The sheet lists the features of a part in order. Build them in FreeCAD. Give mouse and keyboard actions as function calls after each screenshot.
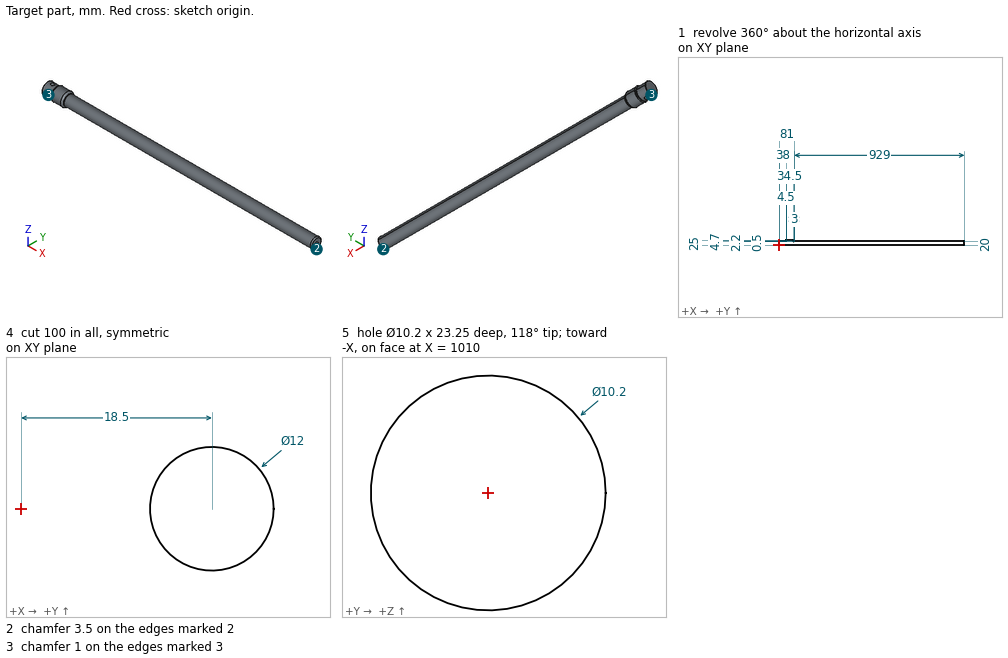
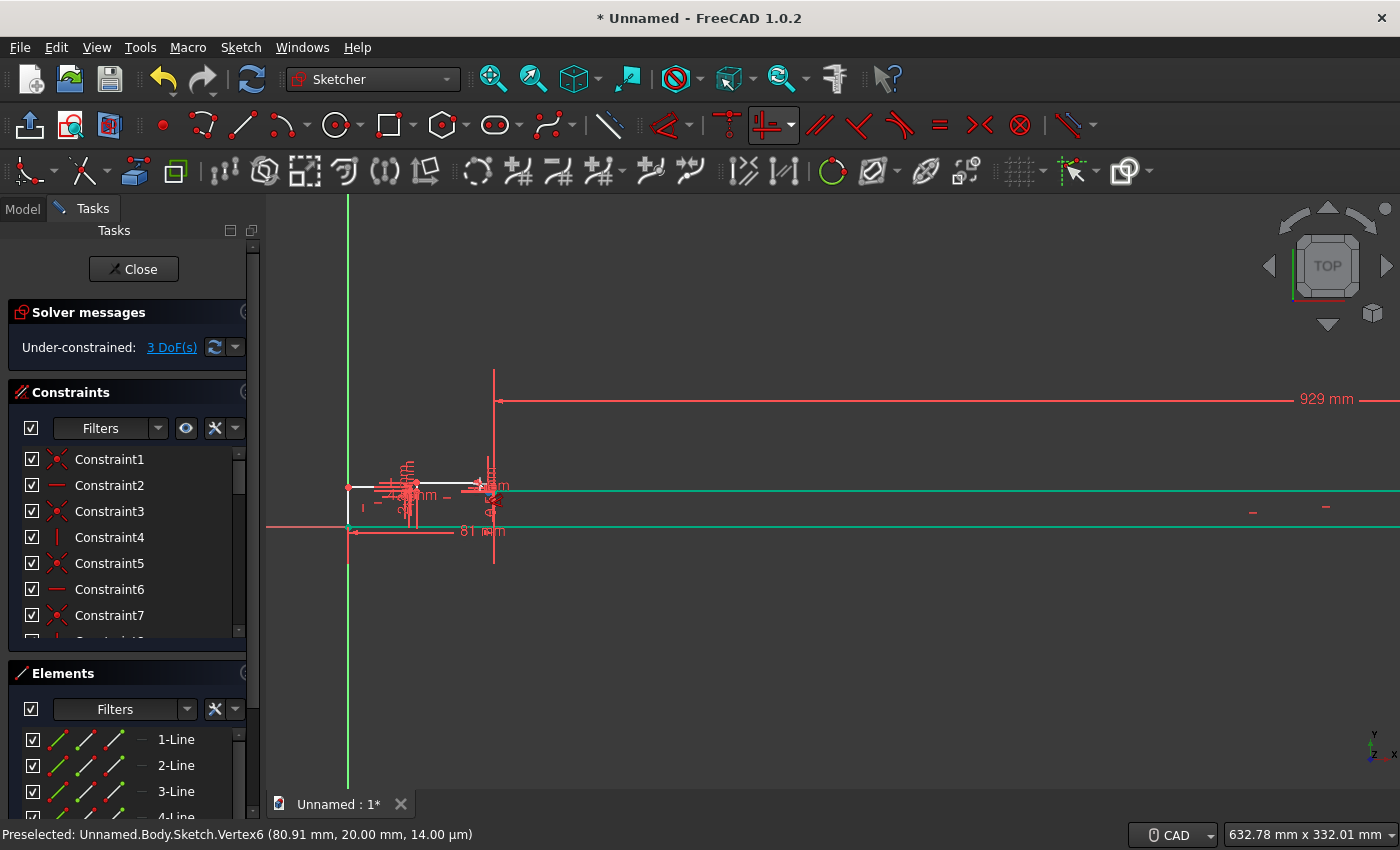
click(478, 483)
click(314, 505)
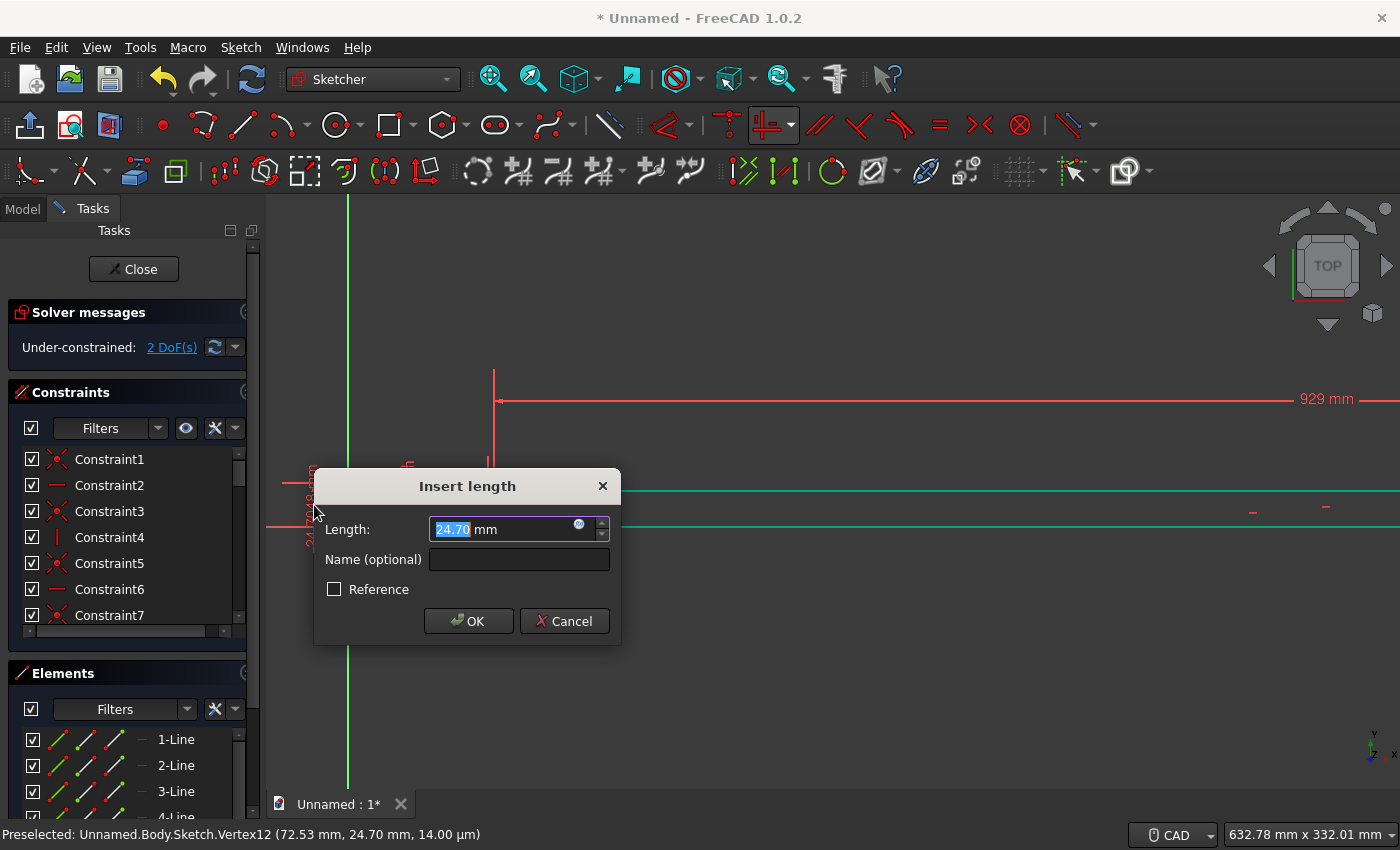
text(25)
key(Return)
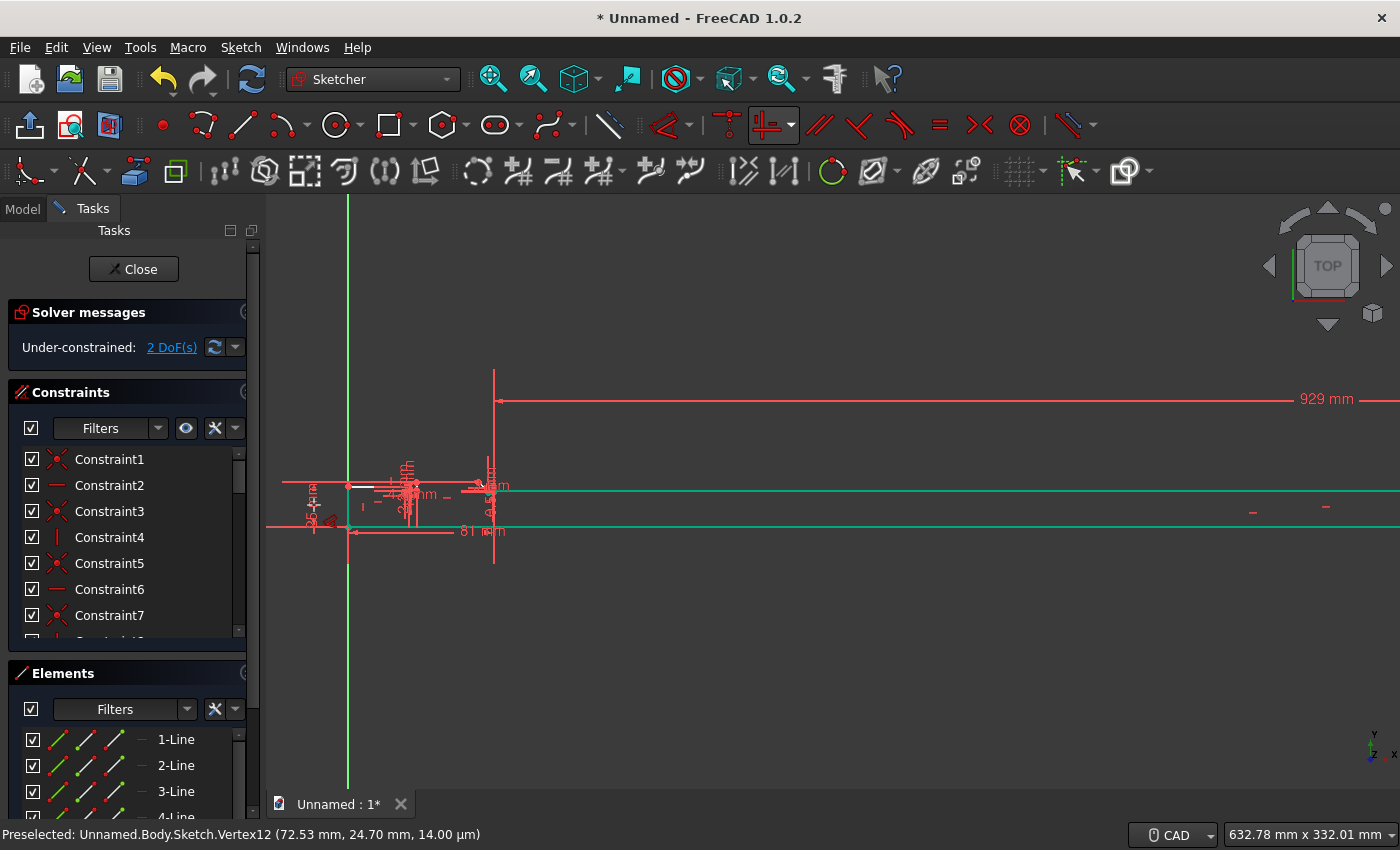
scroll(417, 482, up, 2)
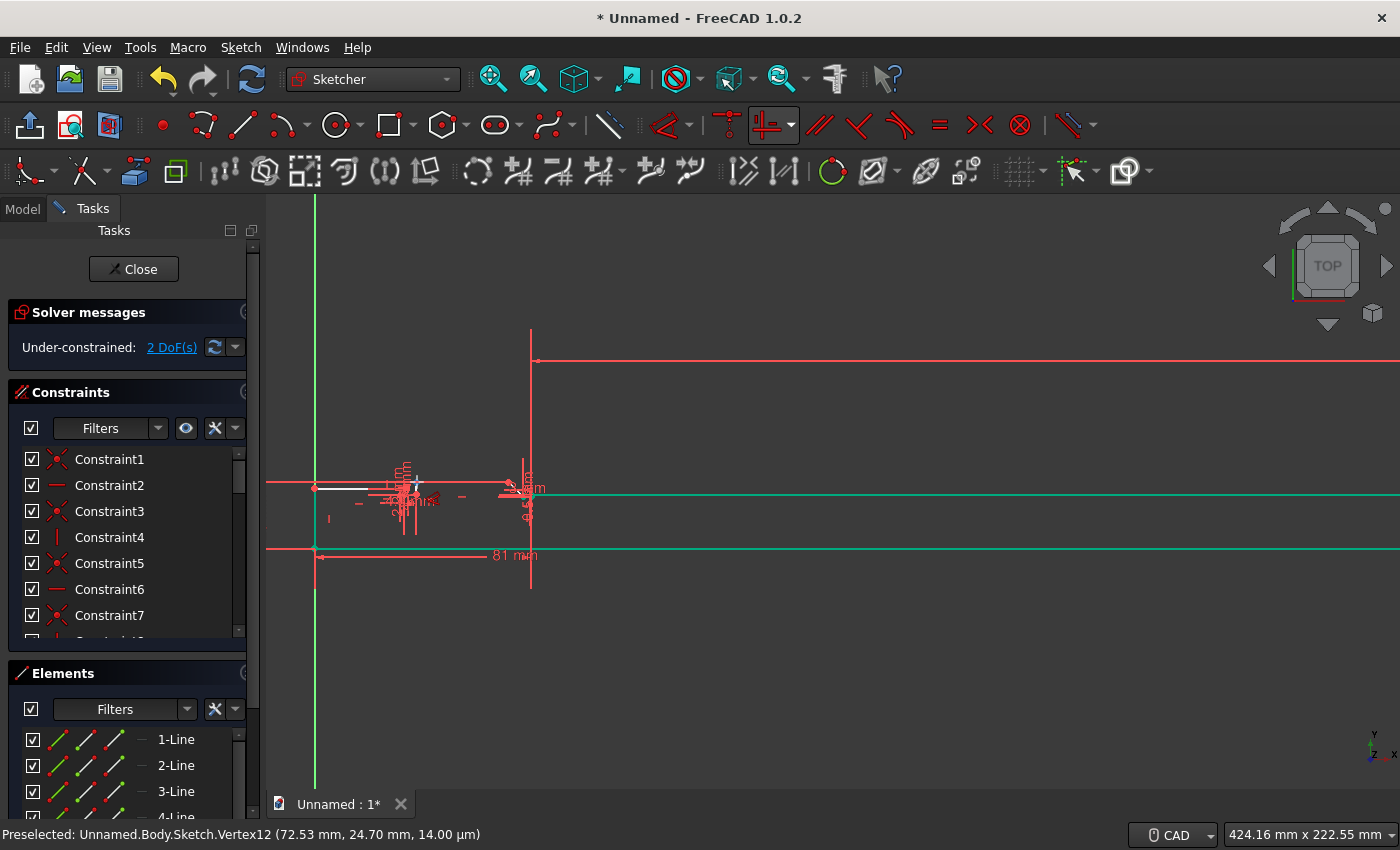
click(416, 482)
click(365, 448)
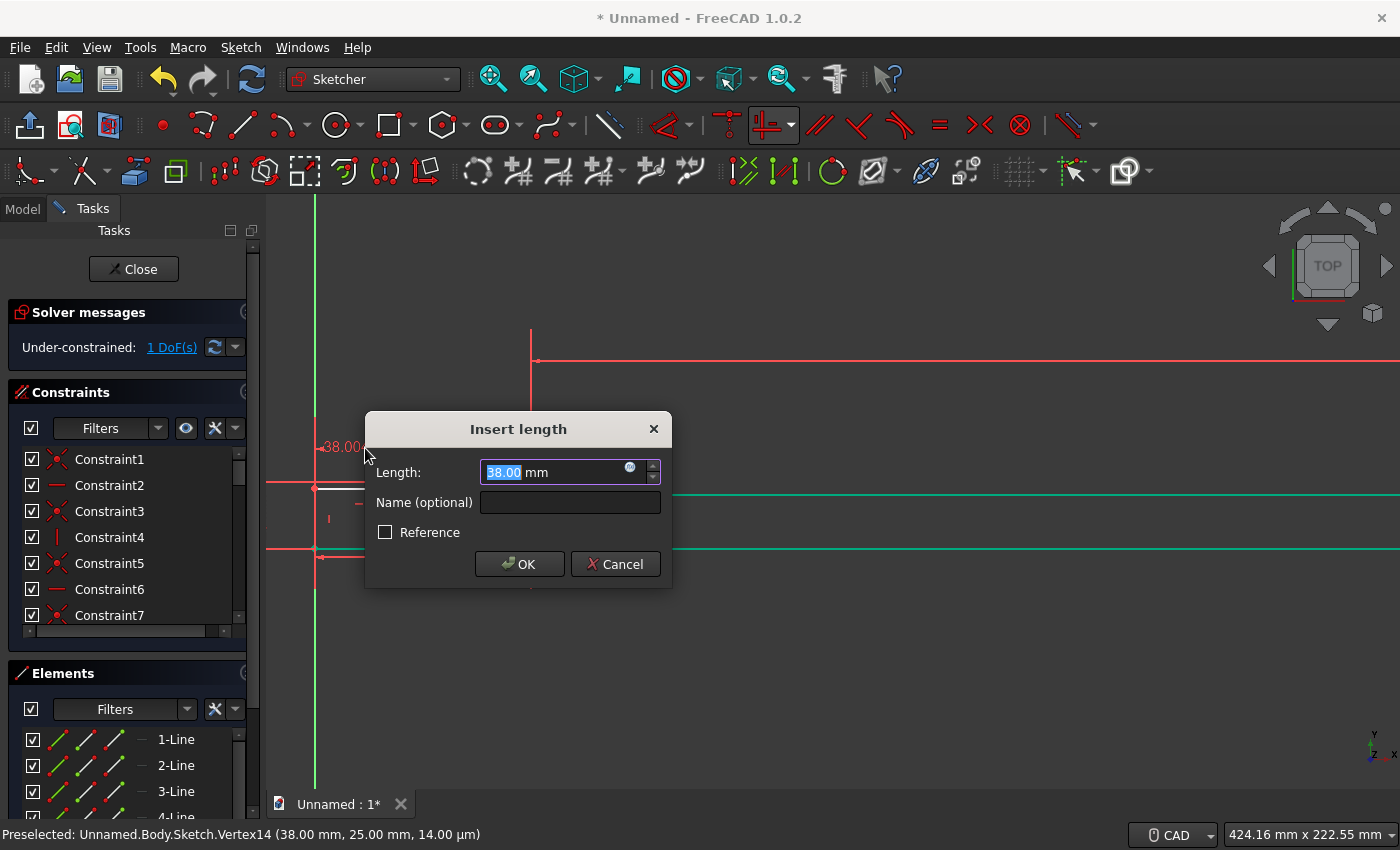
text(38)
key(Return)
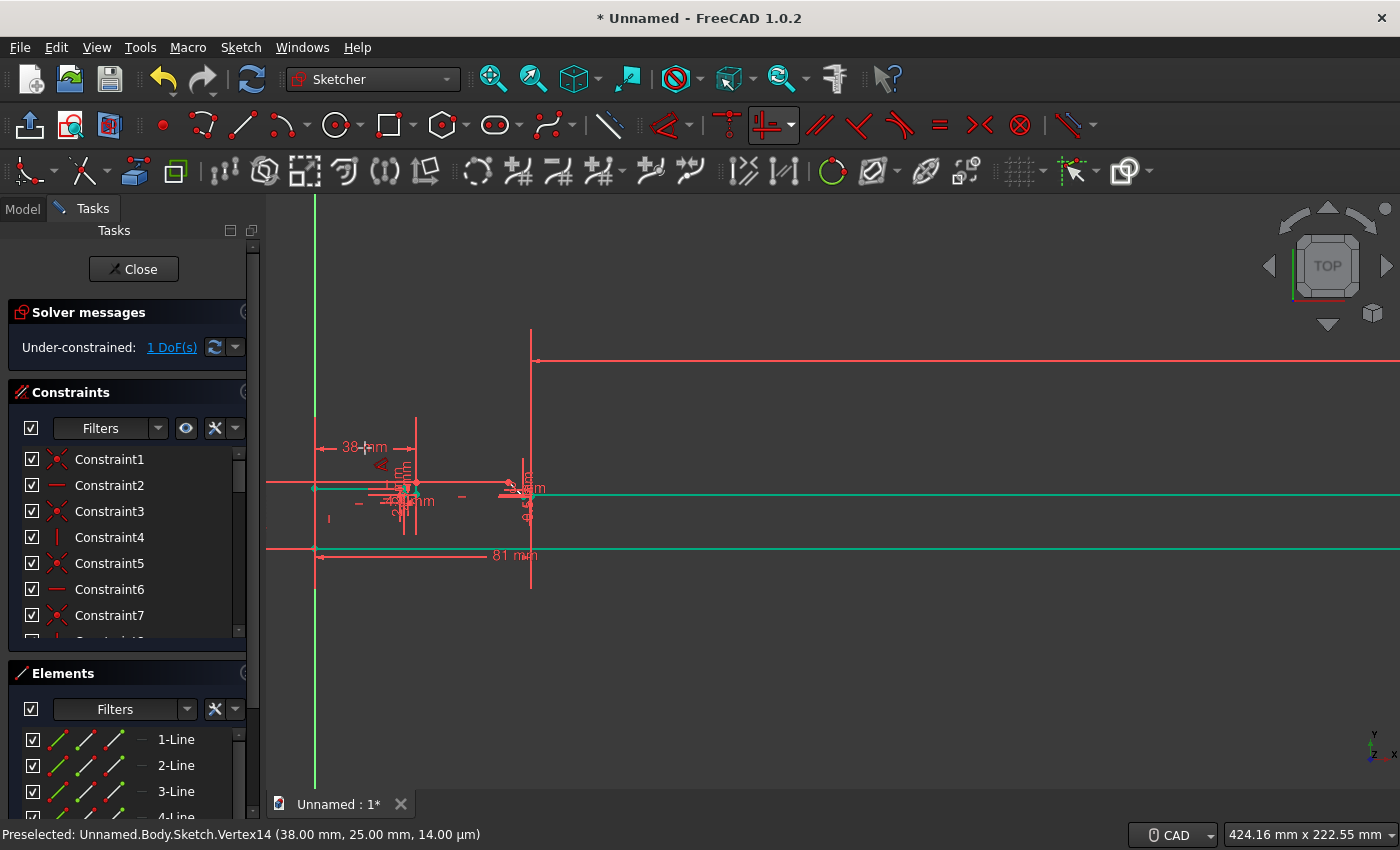
click(481, 482)
click(462, 448)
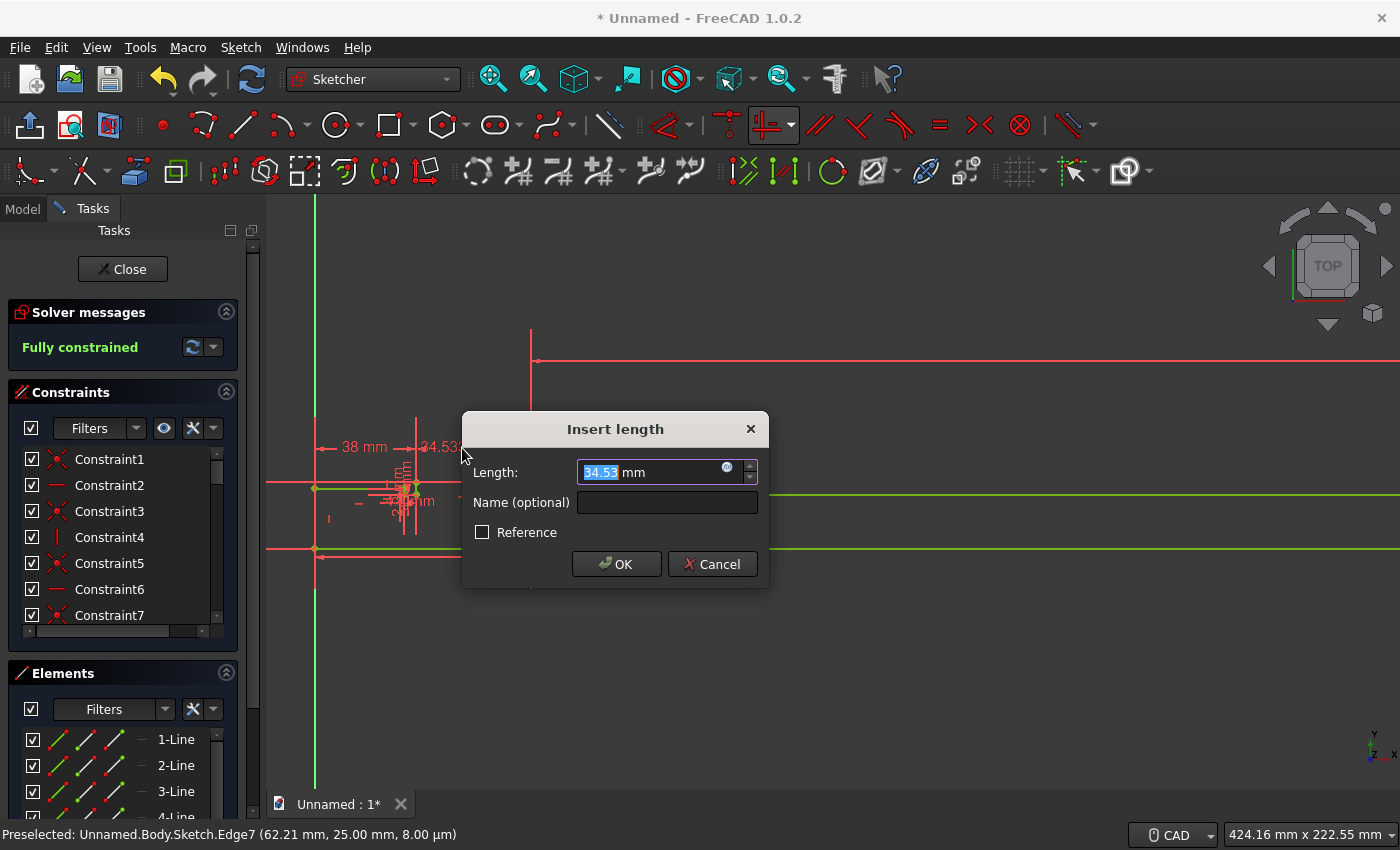
text(34.5)
key(Return)
key(Escape)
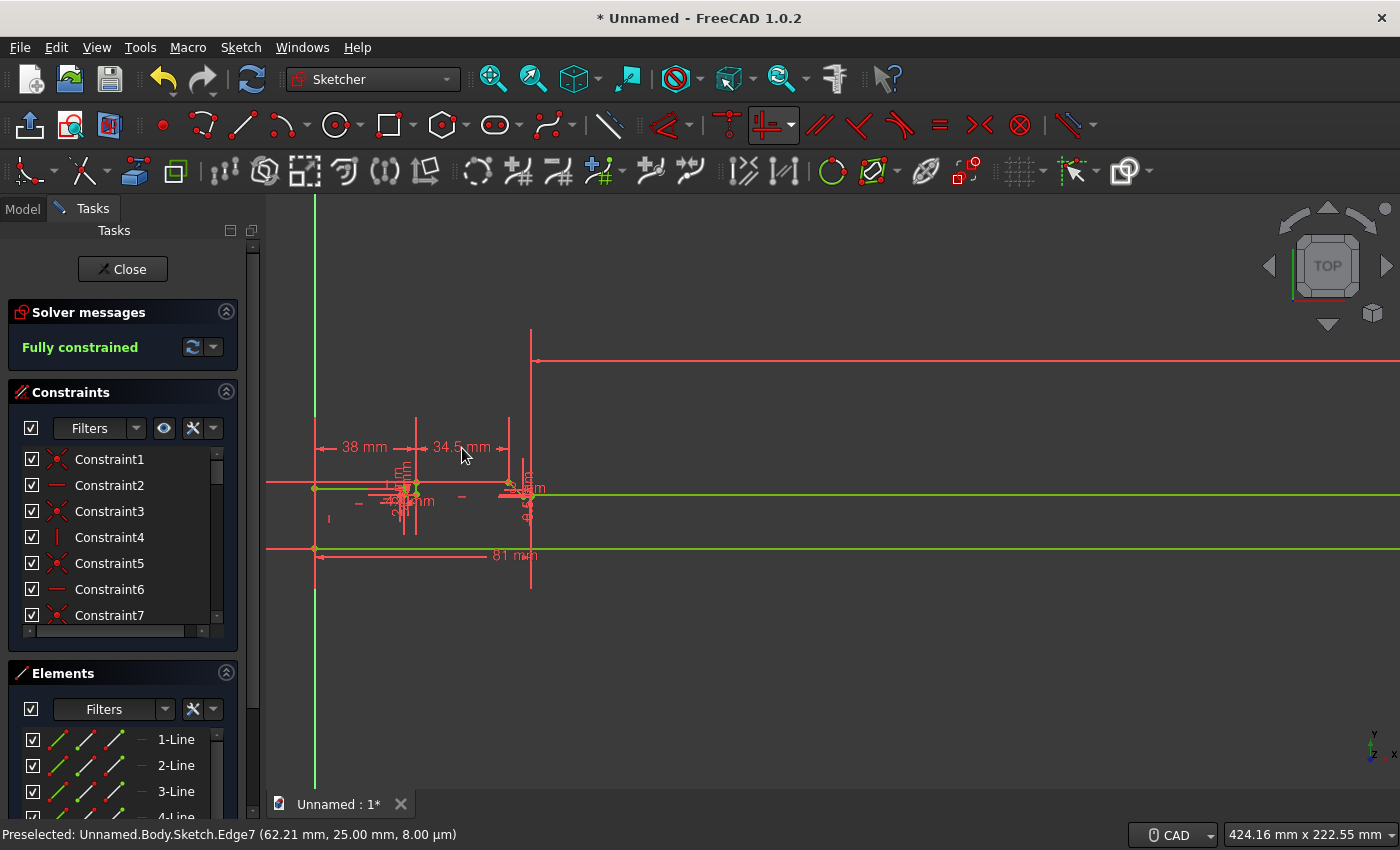
click(123, 269)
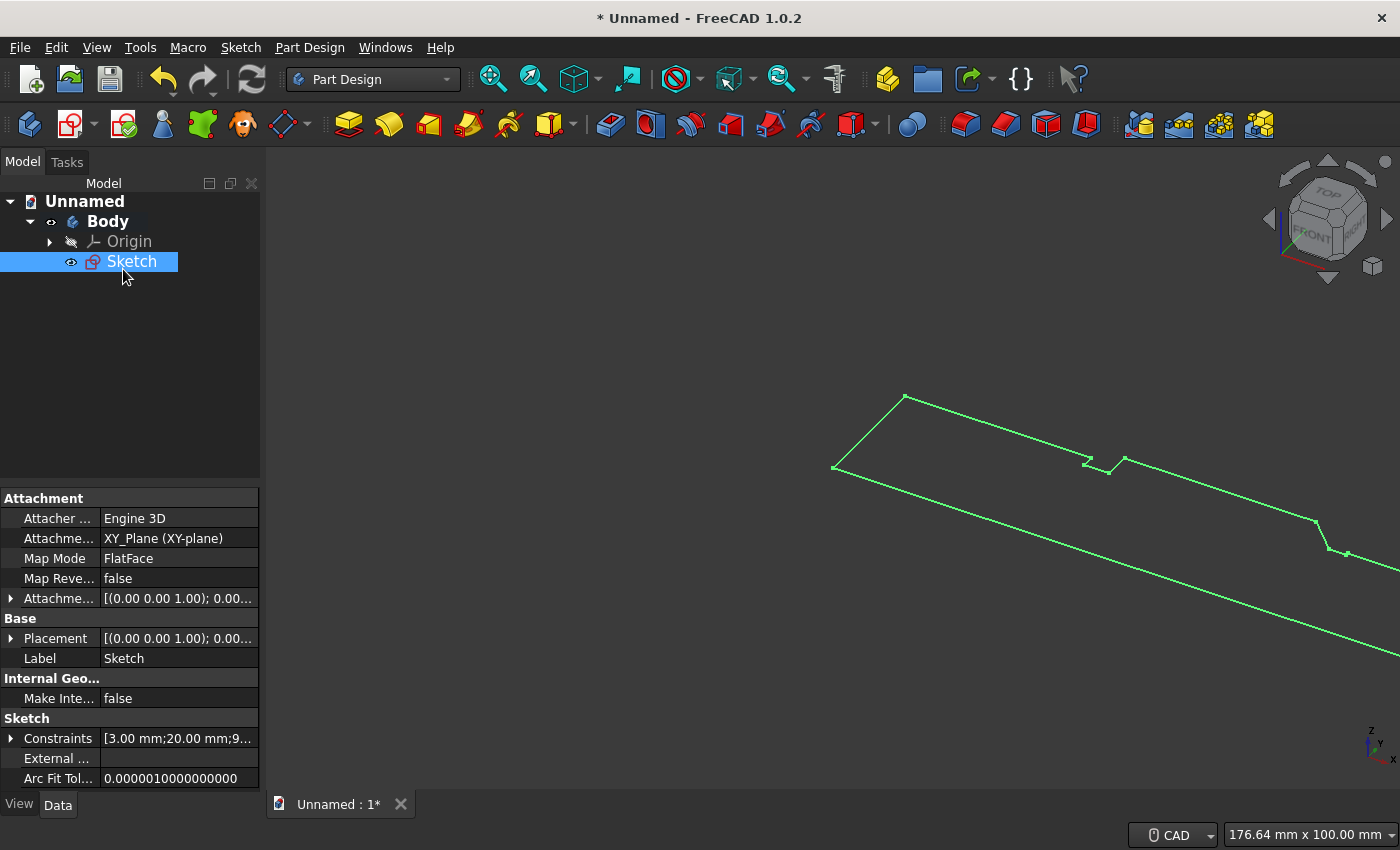
click(390, 124)